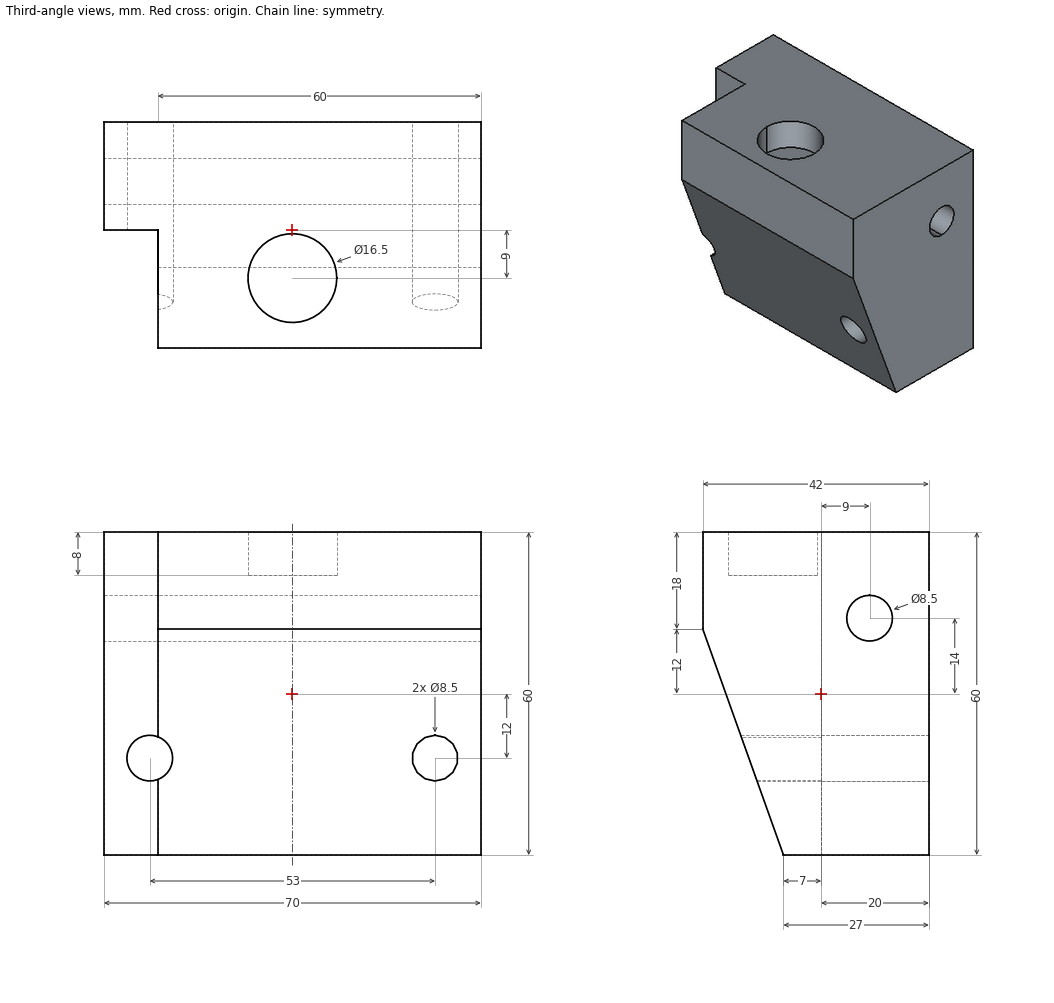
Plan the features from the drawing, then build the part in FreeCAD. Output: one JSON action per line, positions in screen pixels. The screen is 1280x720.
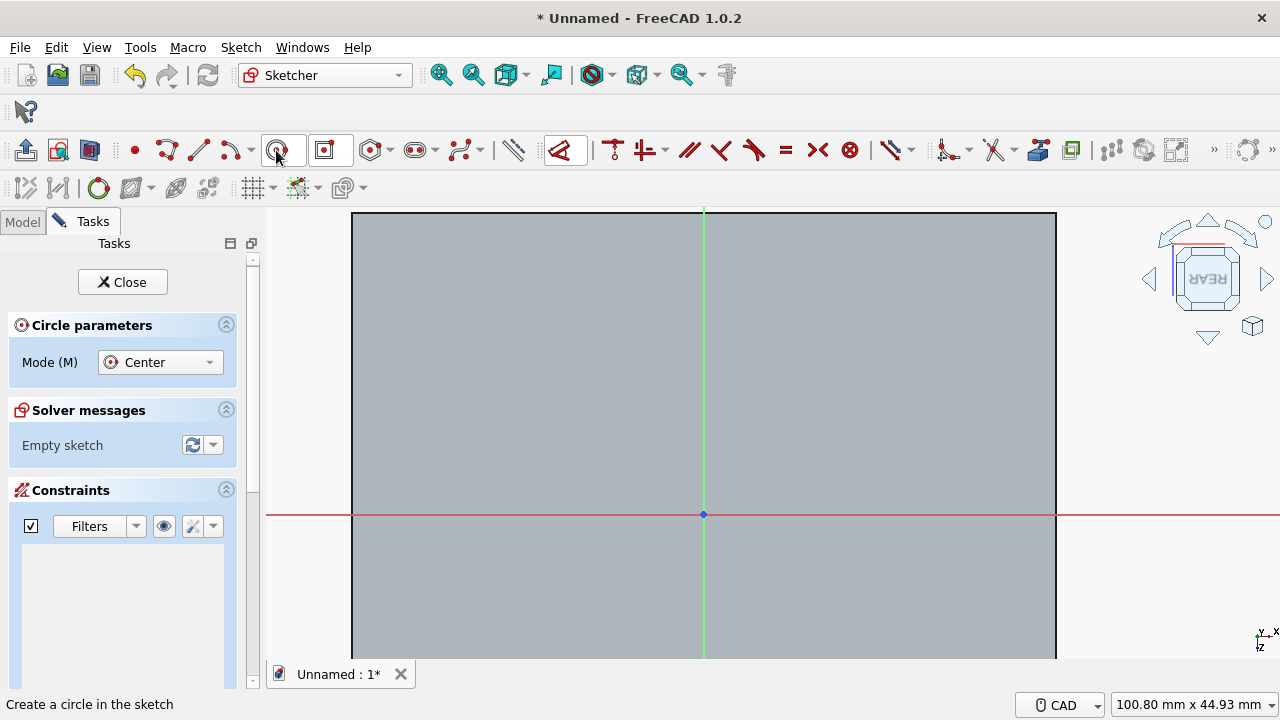
{"action": "left_click", "coordinate": [970, 394]}
{"action": "mouse_move", "coordinate": [1000, 364]}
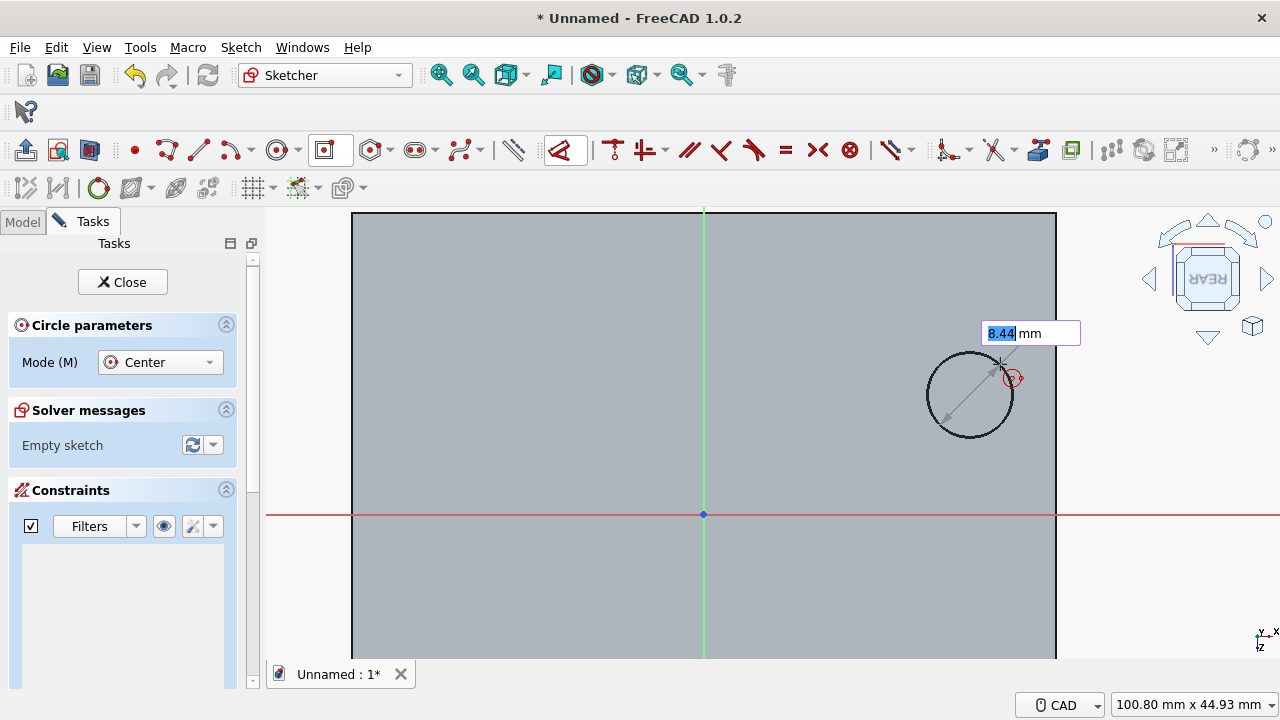
{"action": "type", "text": "8.5"}
{"action": "key", "text": "Return"}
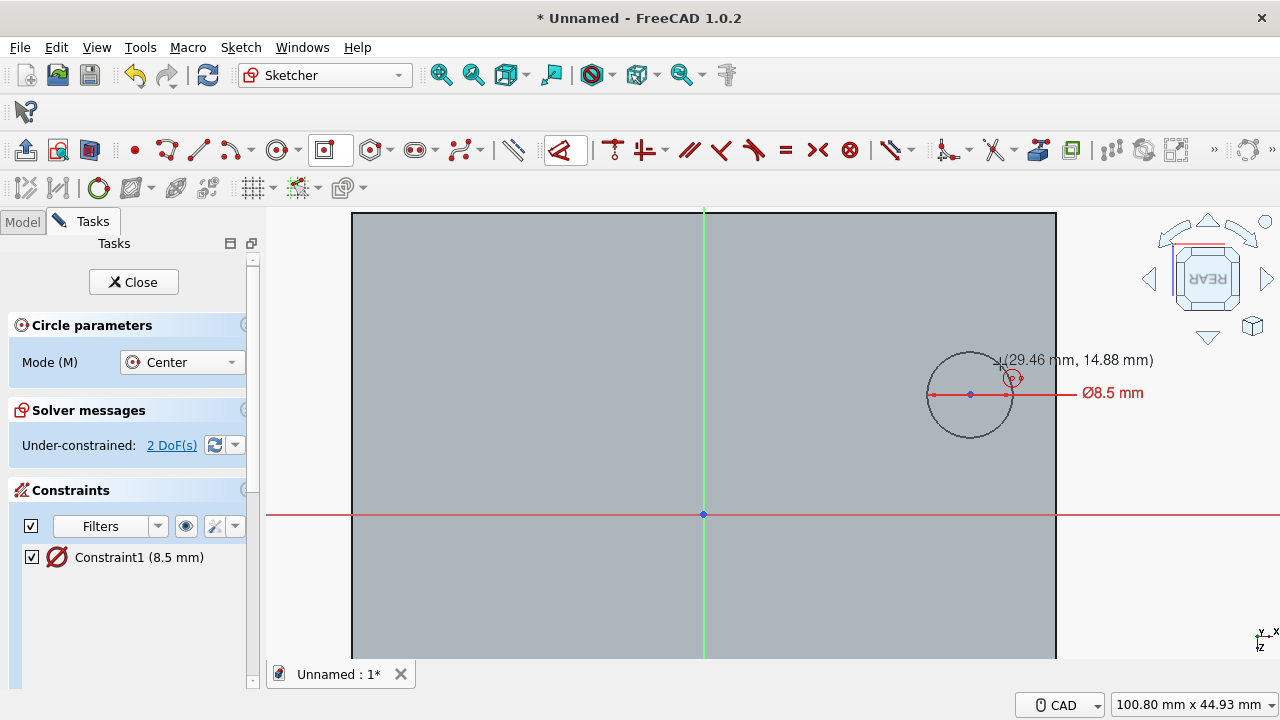
{"action": "left_click", "coordinate": [437, 394]}
{"action": "mouse_move", "coordinate": [467, 364]}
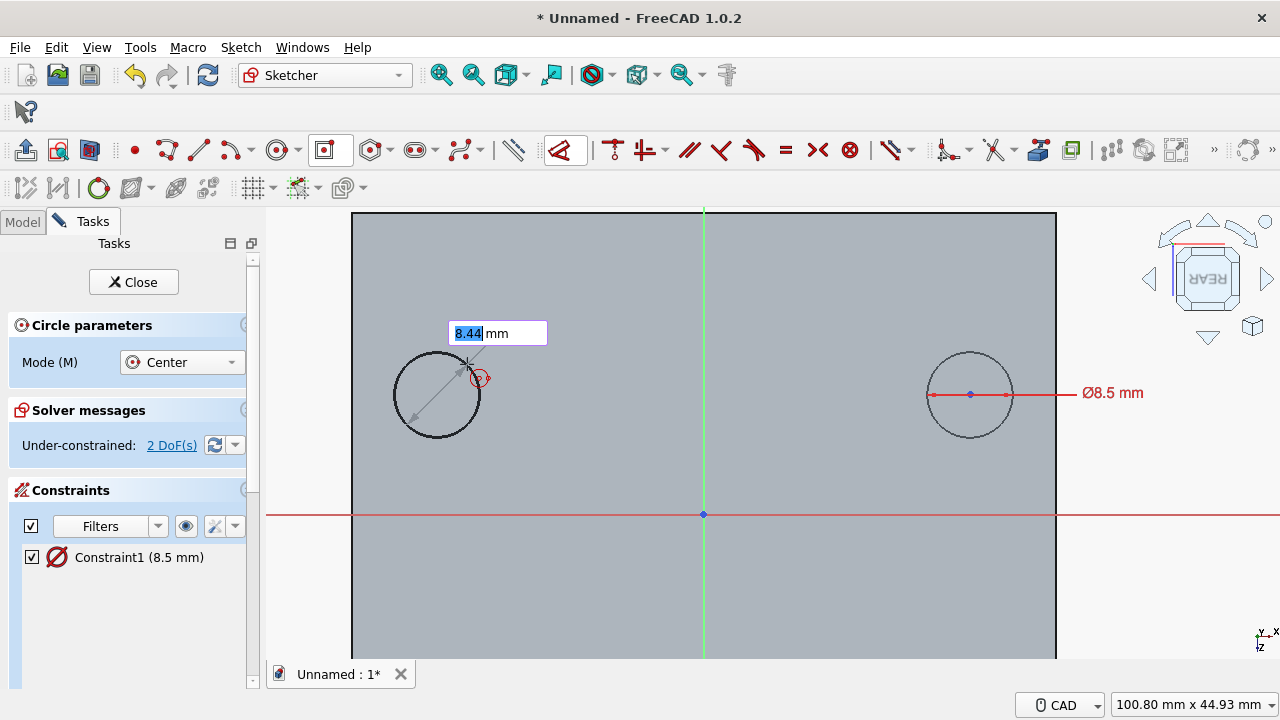
{"action": "type", "text": "8.5"}
{"action": "key", "text": "Return"}
{"action": "key", "text": "Escape"}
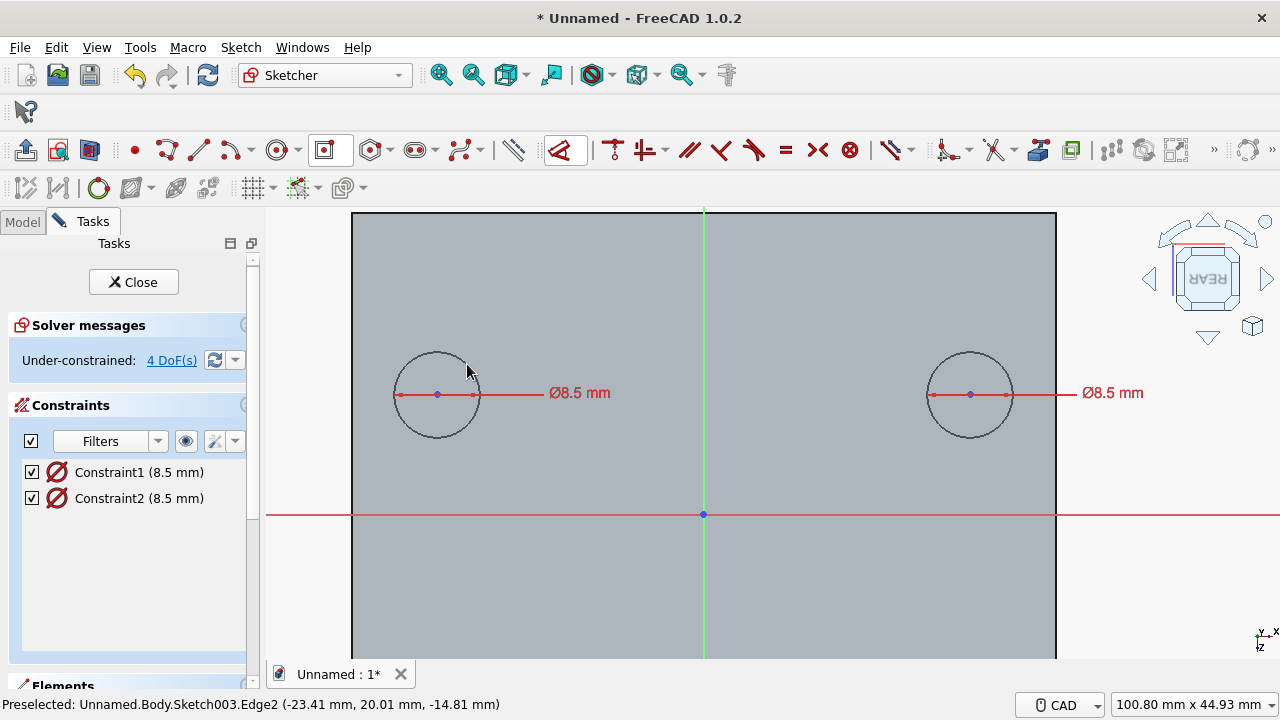
{"action": "left_click", "coordinate": [970, 395]}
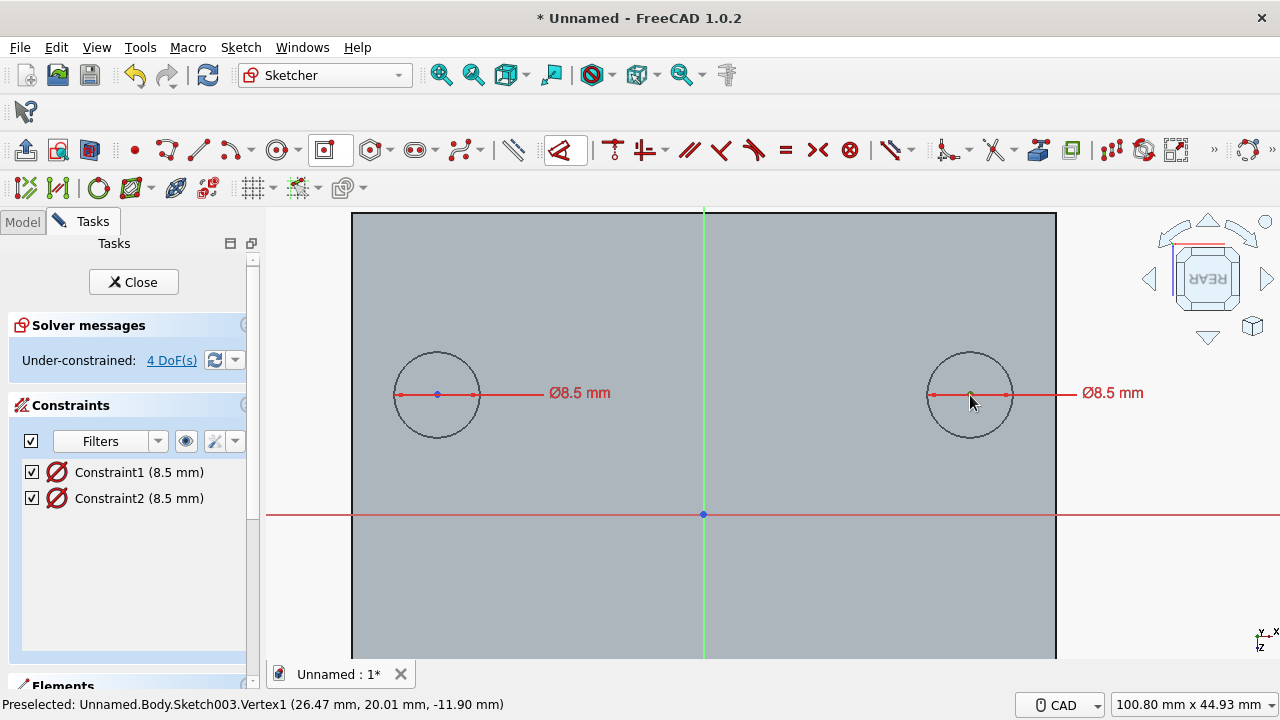
{"action": "left_click", "coordinate": [437, 395]}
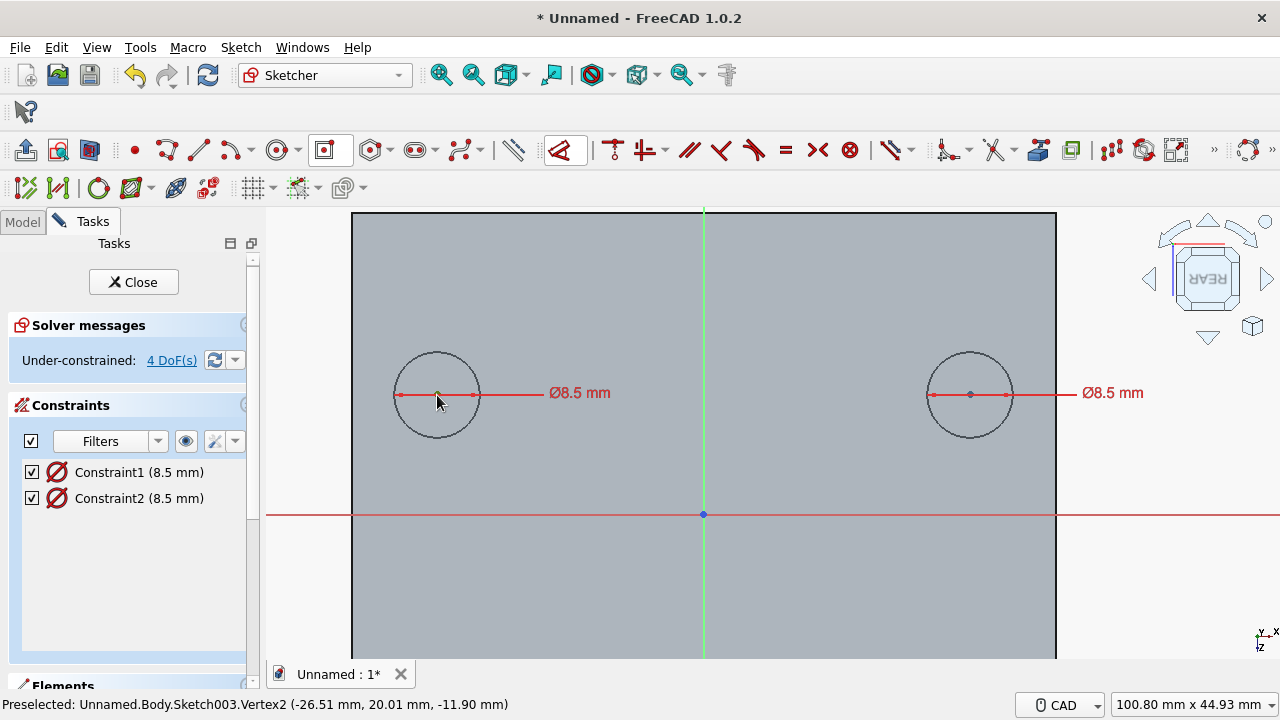
{"action": "left_click", "coordinate": [704, 603]}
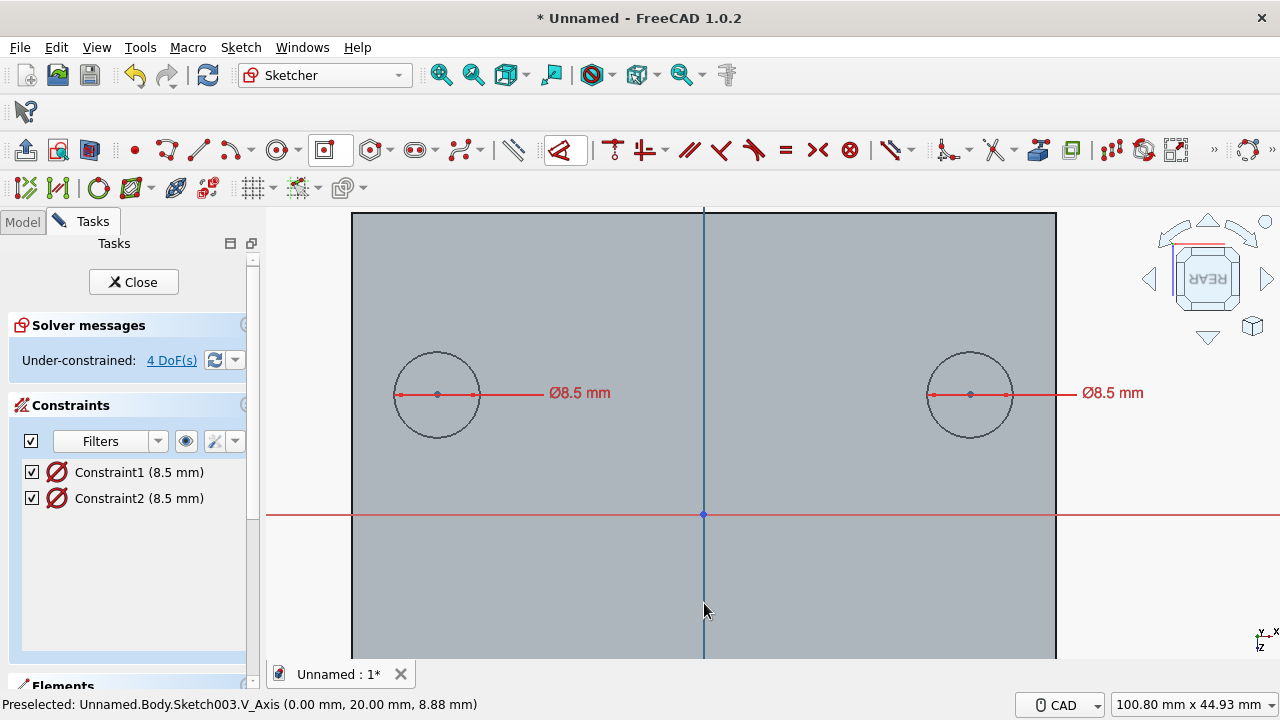
{"action": "key", "text": "s"}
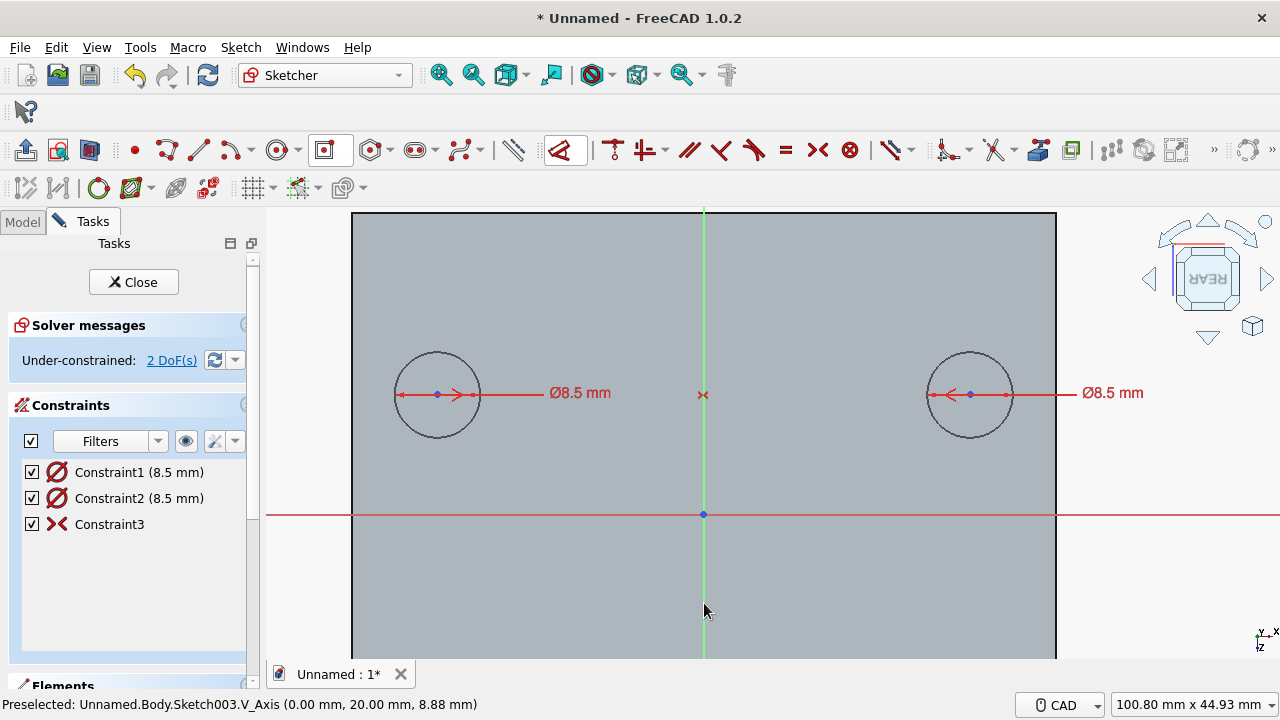
{"action": "left_click", "coordinate": [970, 395]}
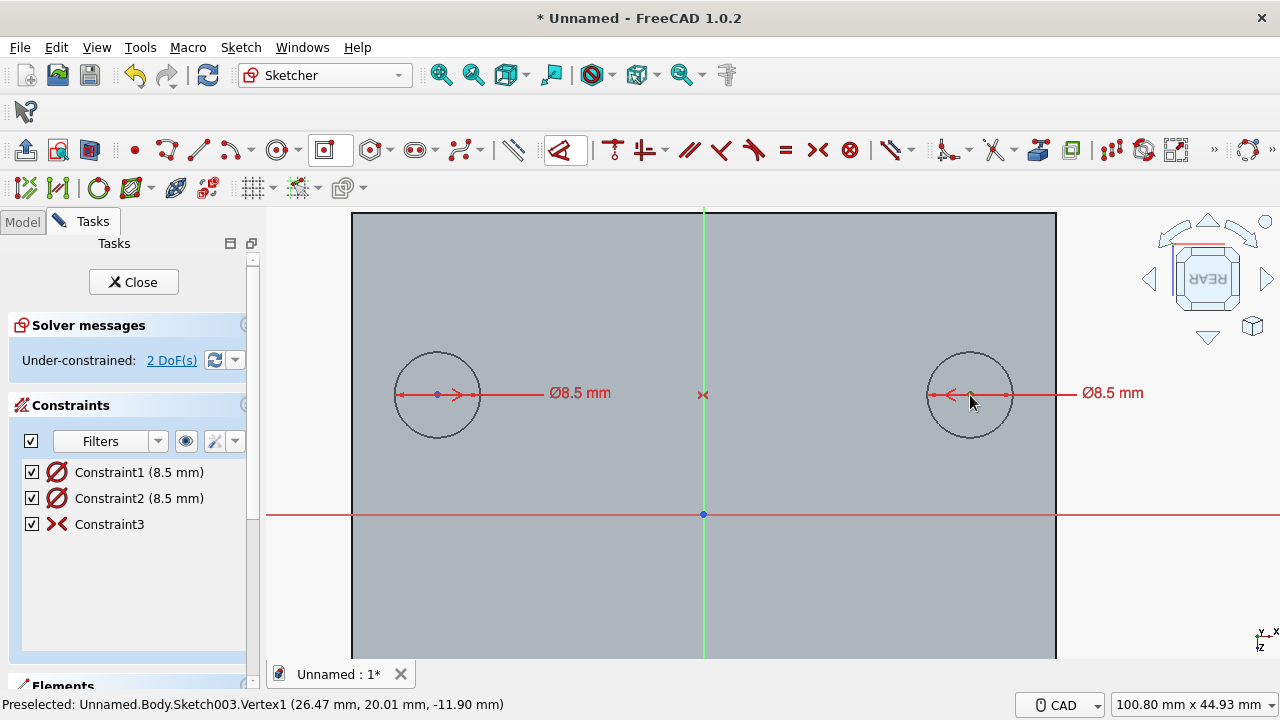
{"action": "key", "text": "i"}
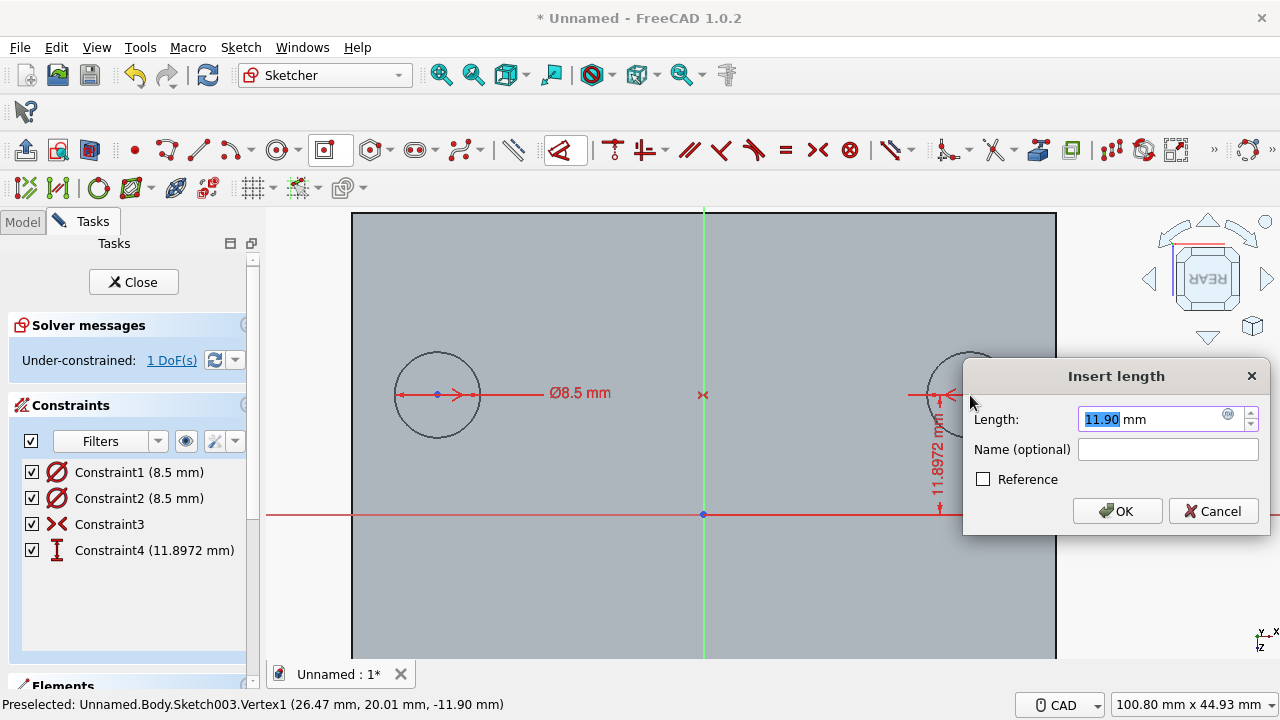
{"action": "type", "text": "12"}
{"action": "key", "text": "Return"}